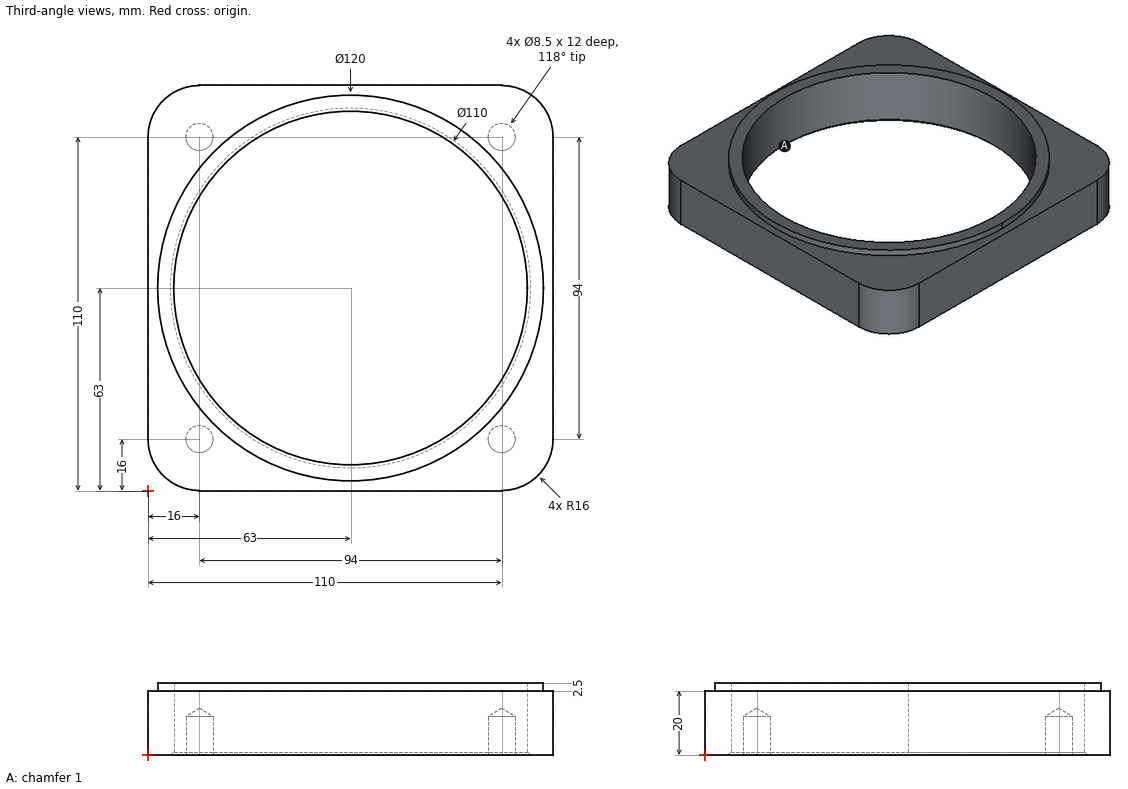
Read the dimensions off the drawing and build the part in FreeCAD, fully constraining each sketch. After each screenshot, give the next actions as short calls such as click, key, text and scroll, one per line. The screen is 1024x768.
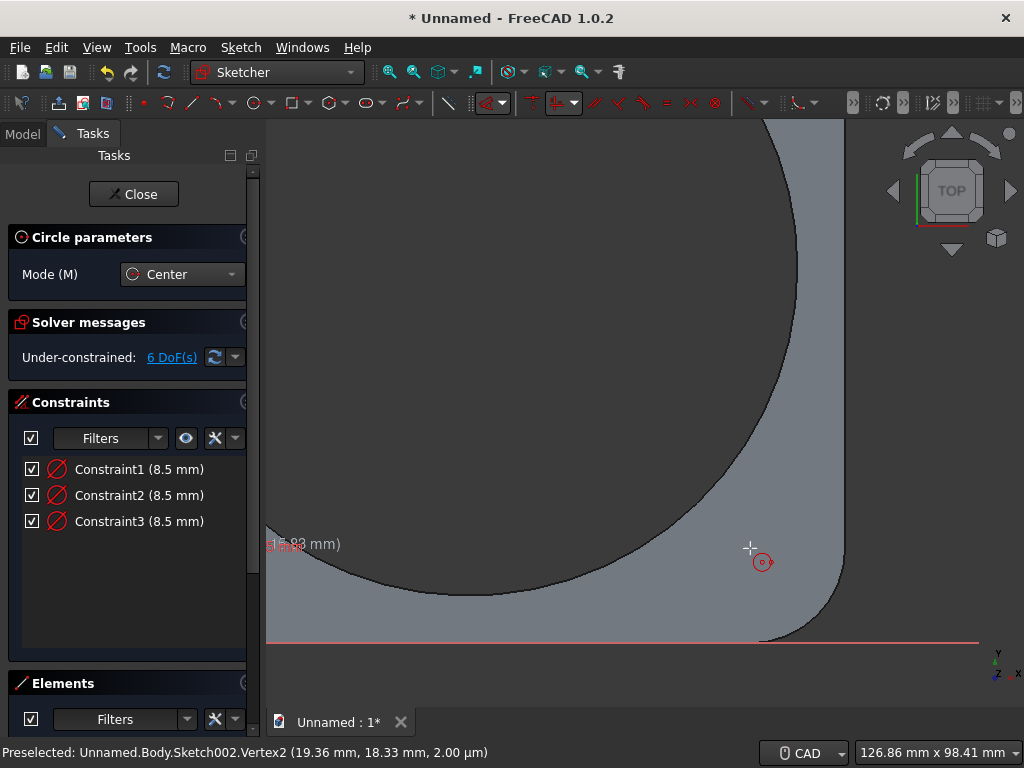
click(750, 548)
move(768, 530)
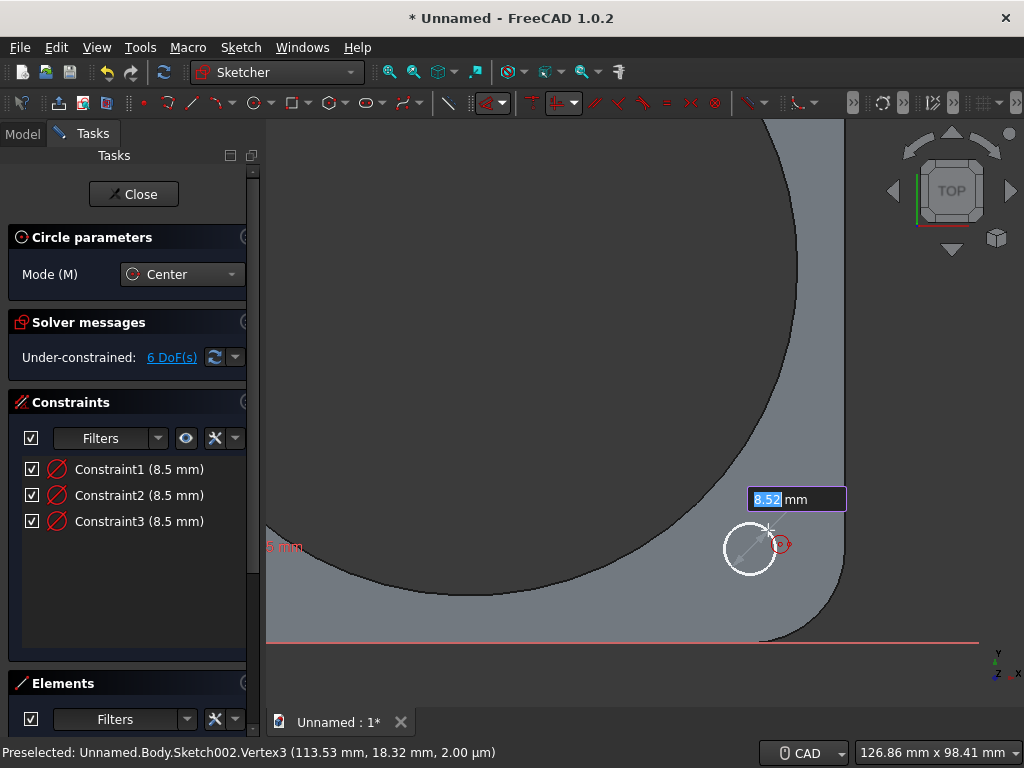
text(8.5)
key(Return)
key(Escape)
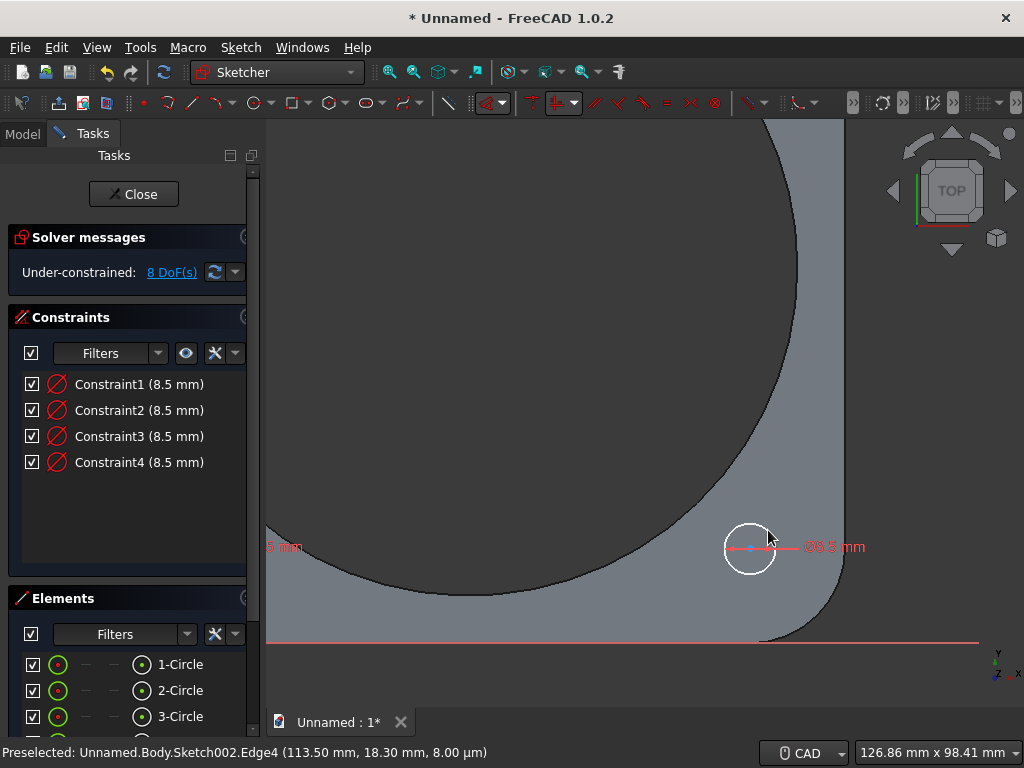
scroll(750, 548, down, 3)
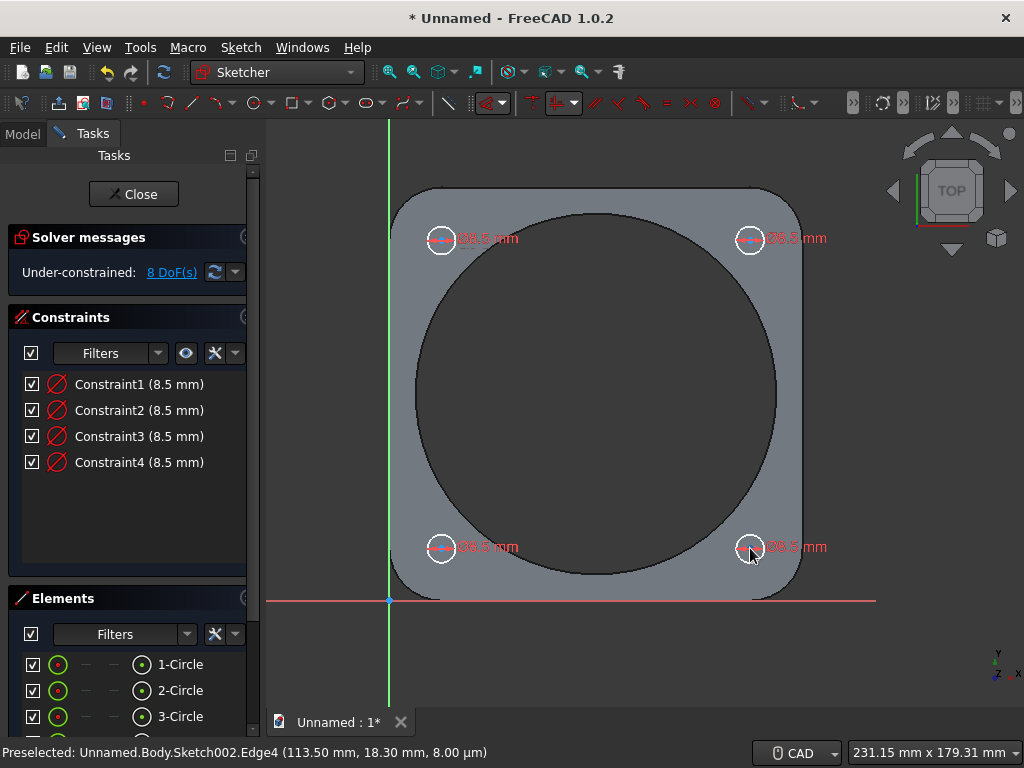
click(442, 241)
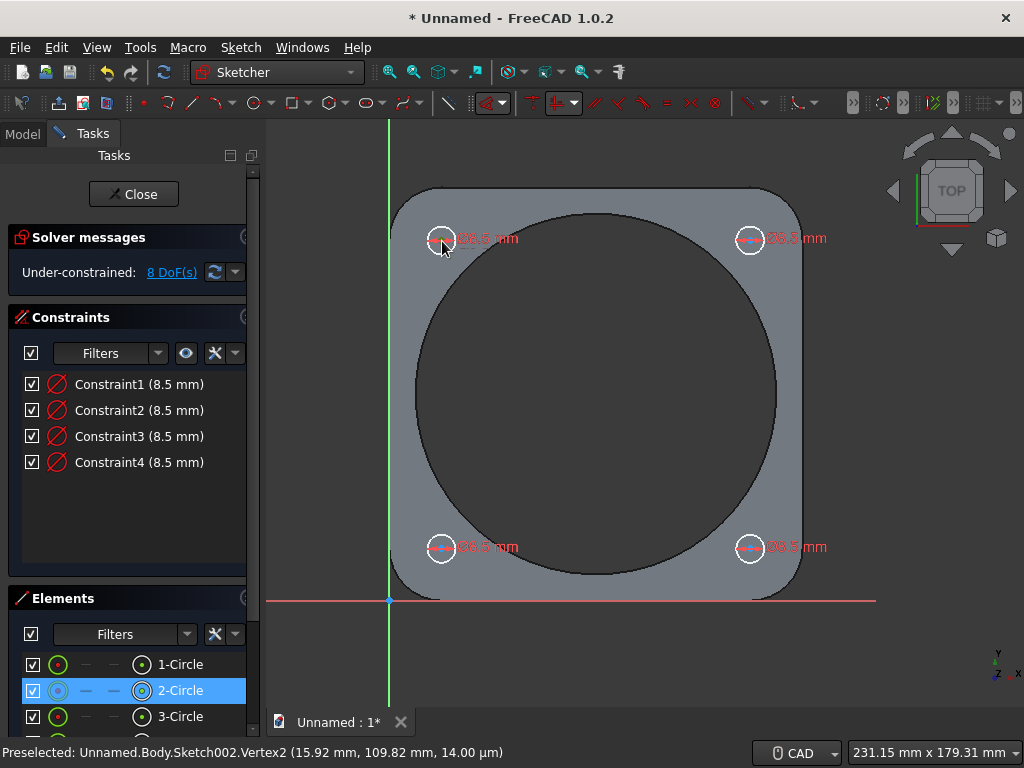
click(504, 104)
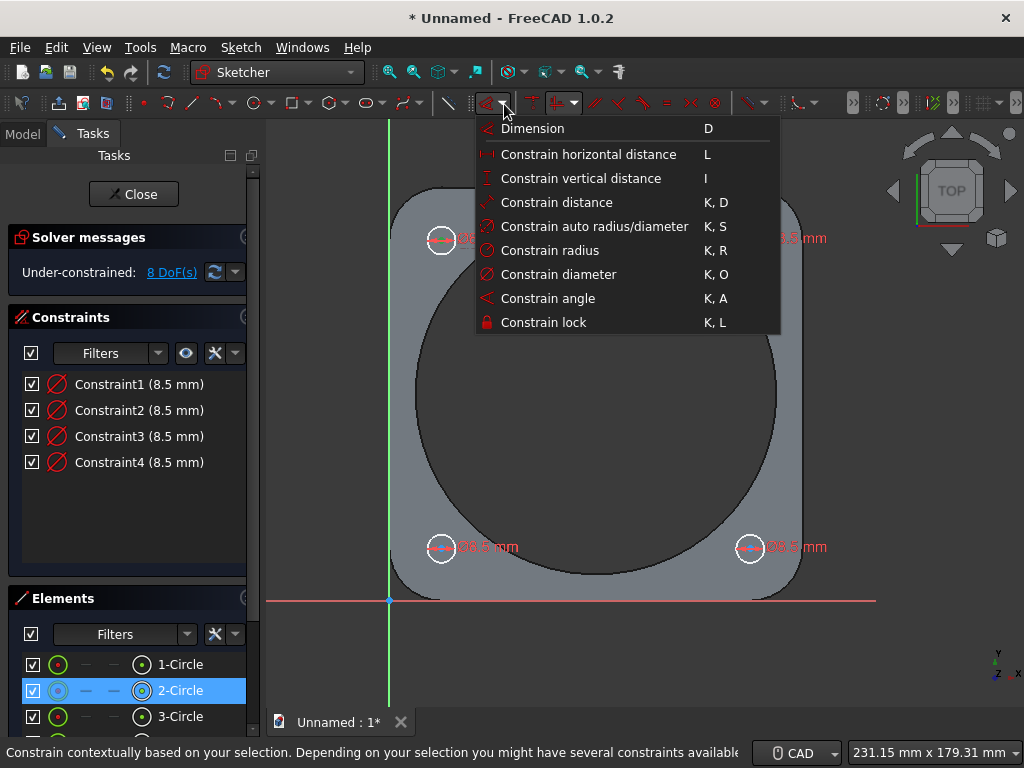
click(628, 154)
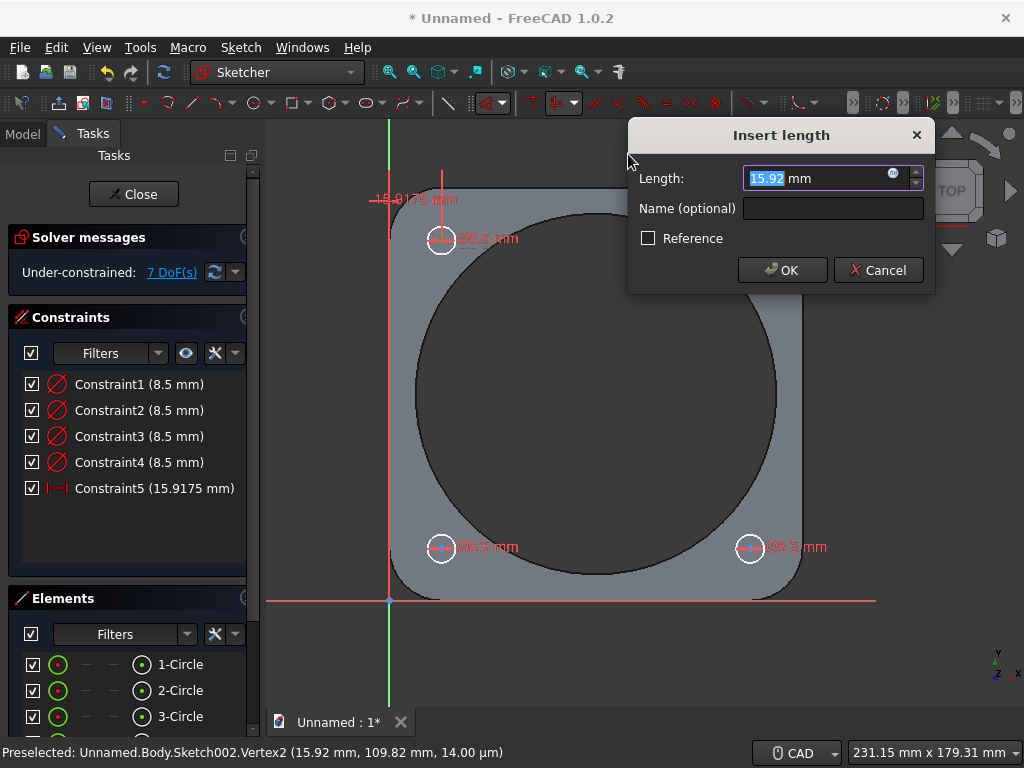
text(16)
key(Return)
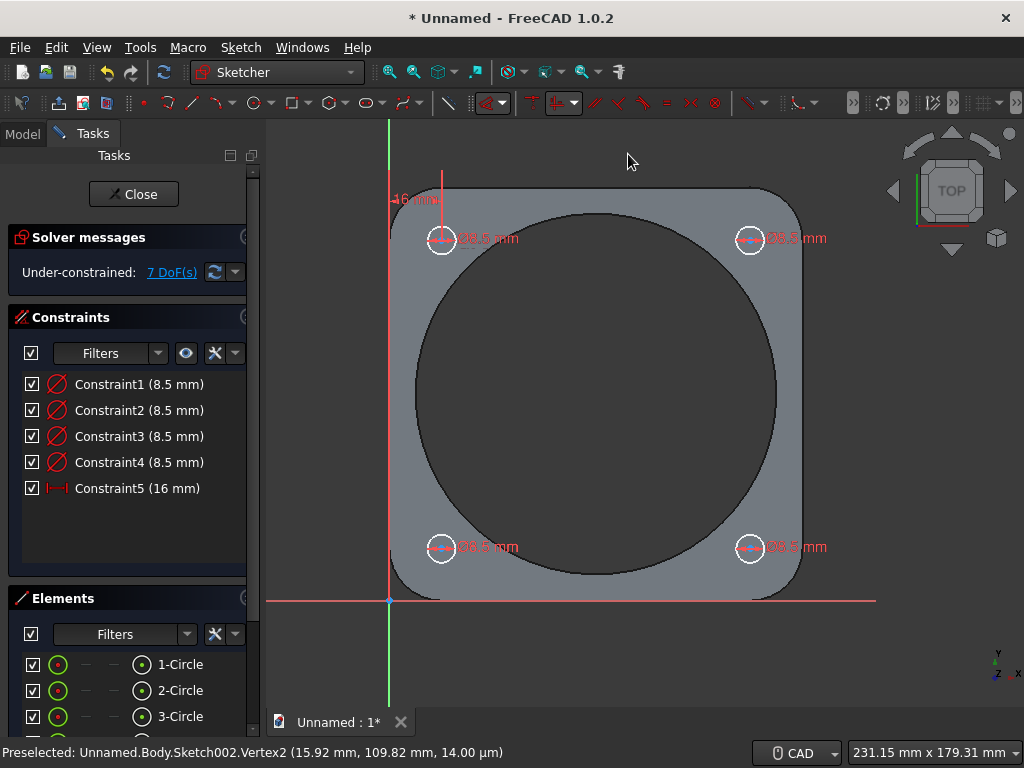
click(442, 549)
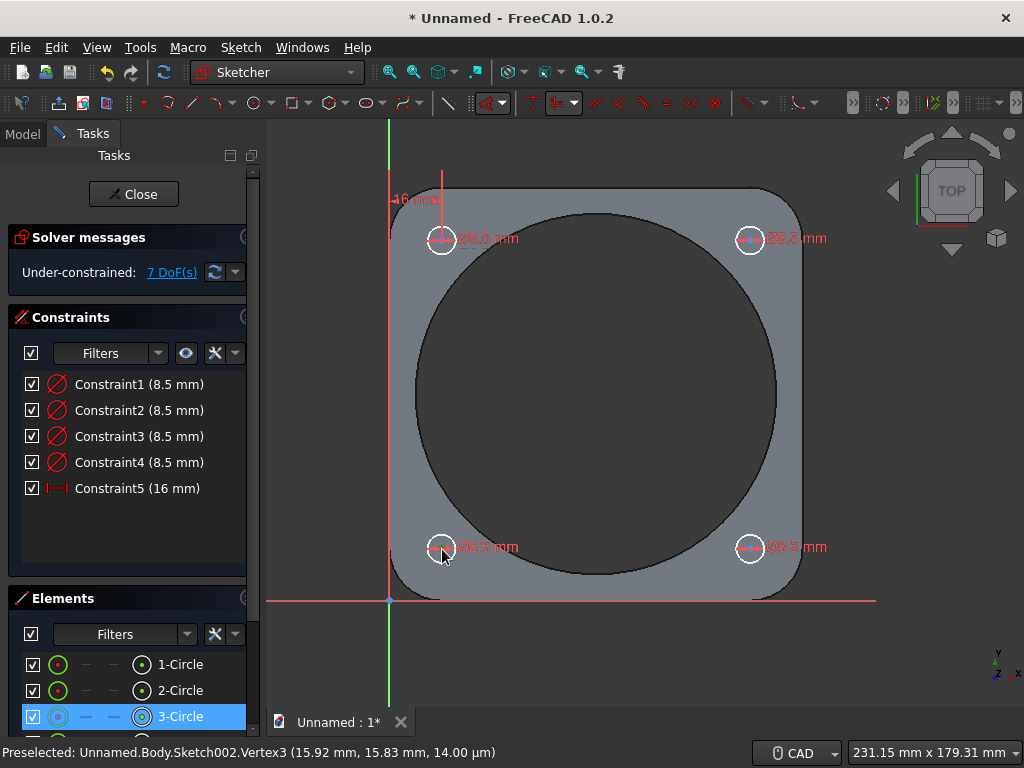
click(504, 104)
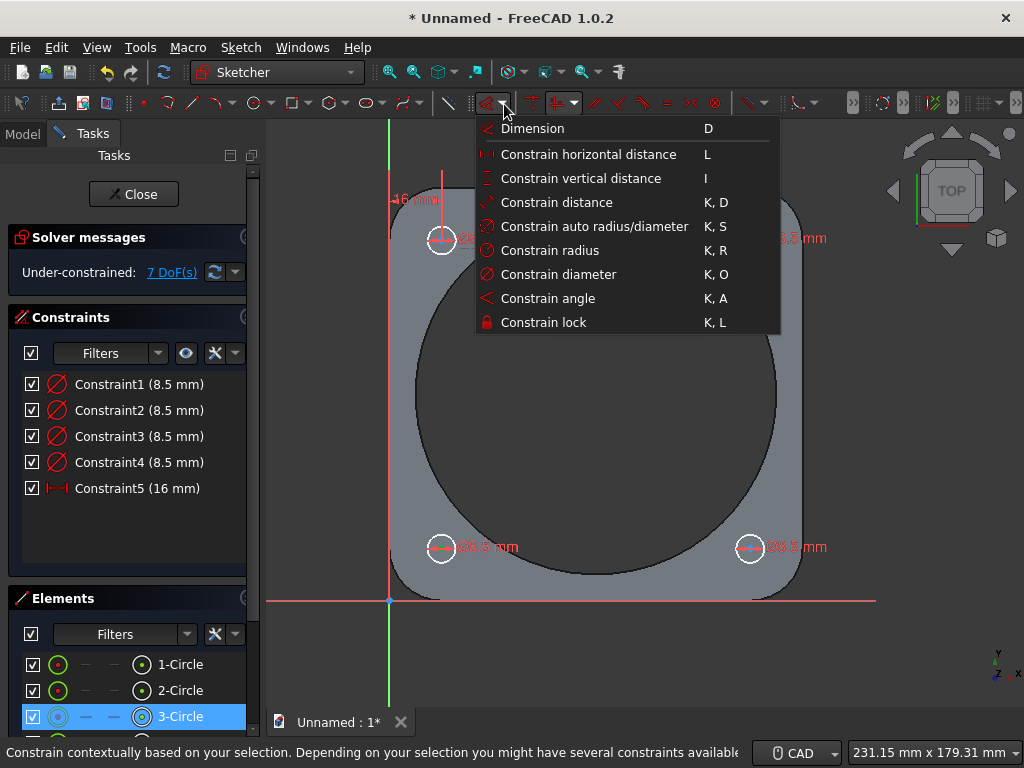
click(628, 154)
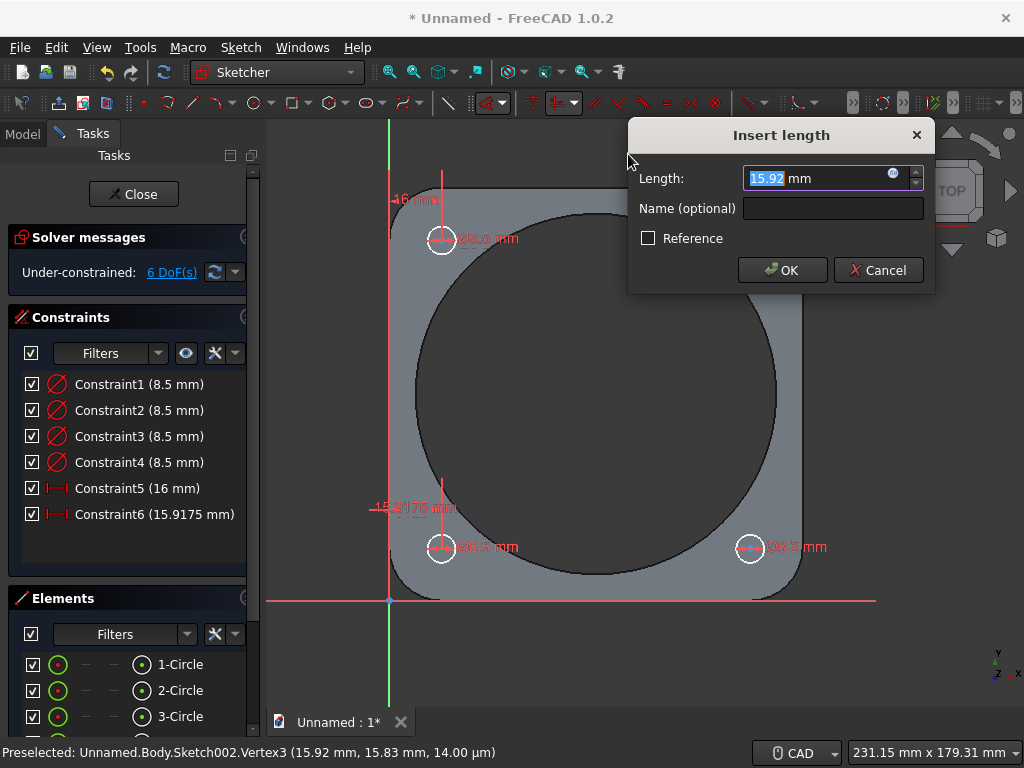
text(16)
key(Return)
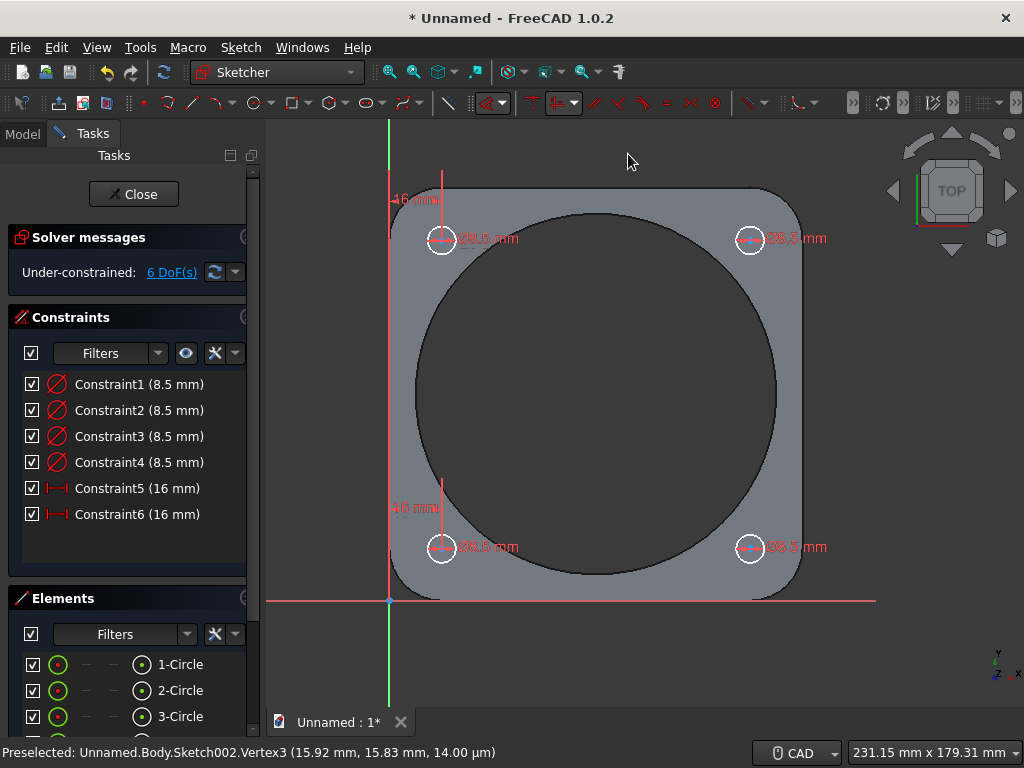
click(442, 549)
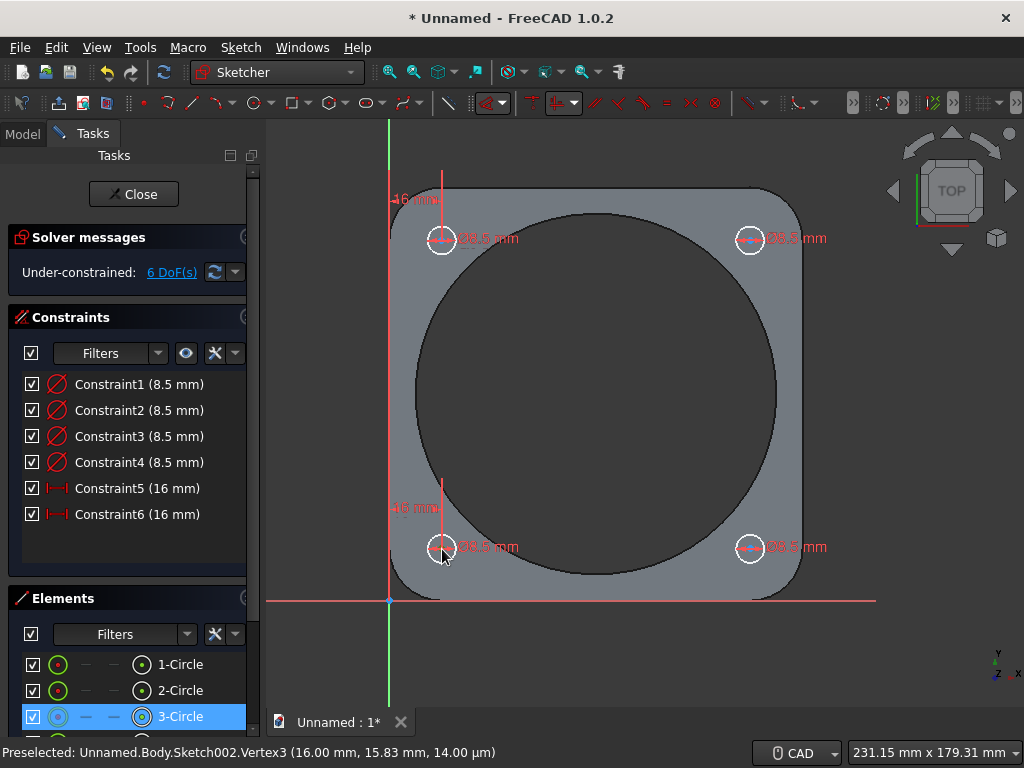
key(i)